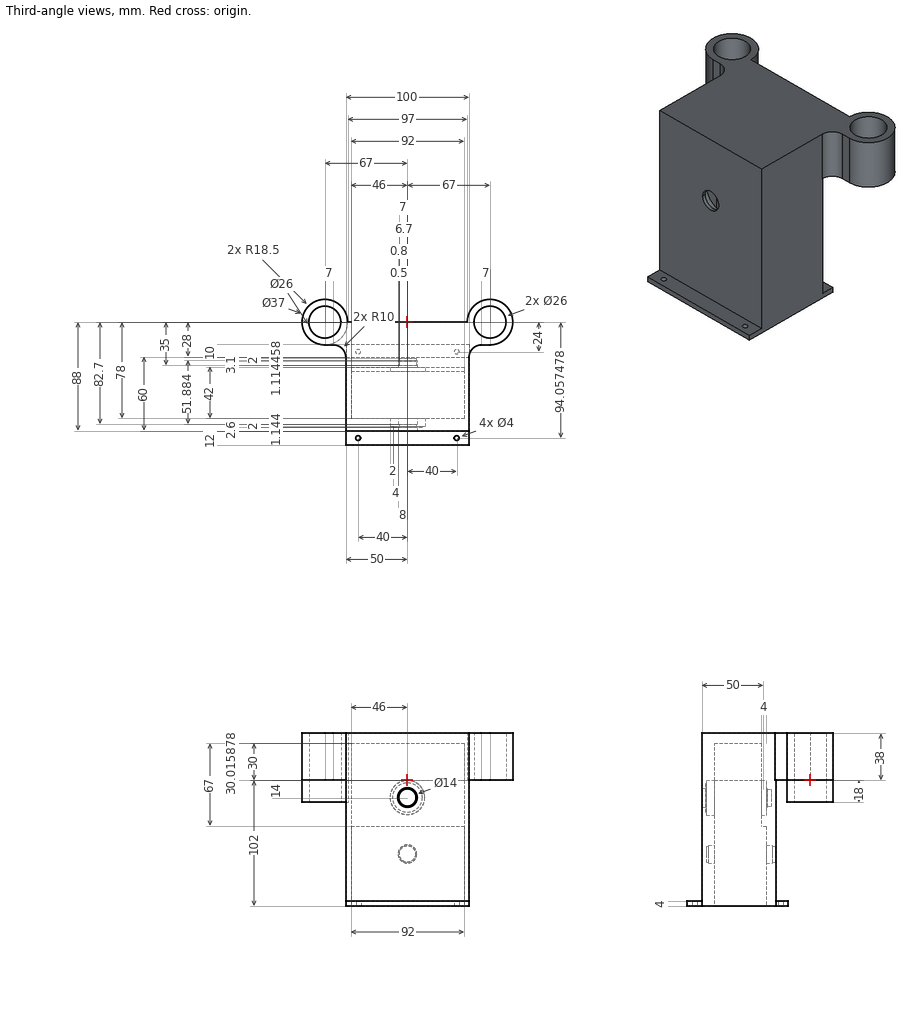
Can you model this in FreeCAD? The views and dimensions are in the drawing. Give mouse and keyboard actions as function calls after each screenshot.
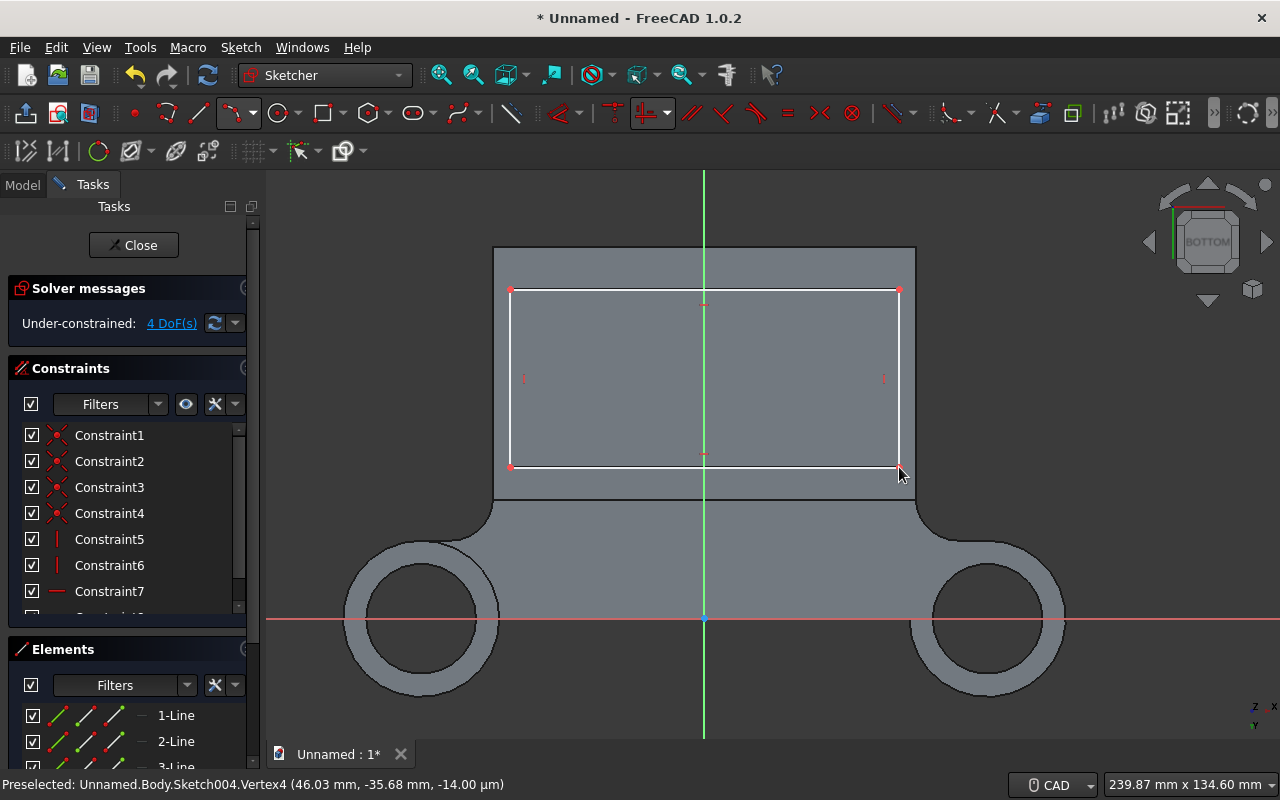
key(d)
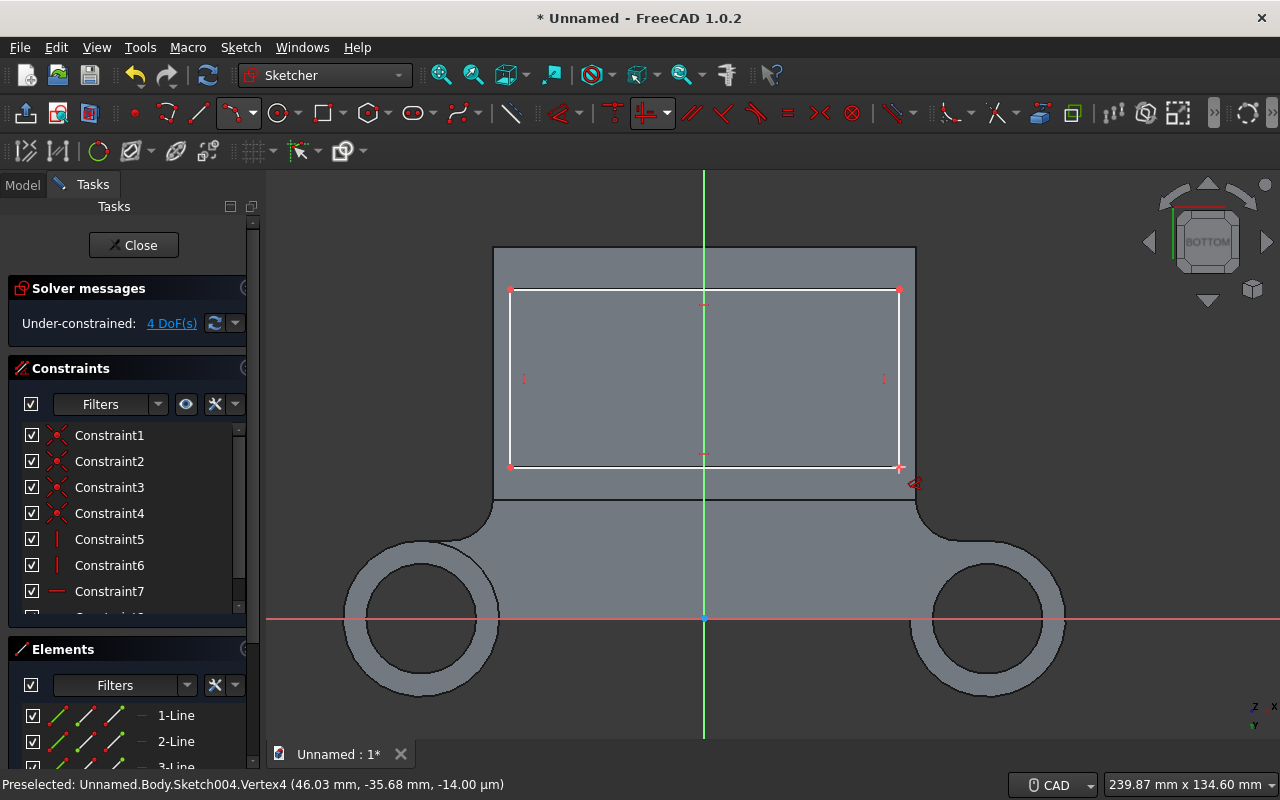
click(510, 343)
click(476, 379)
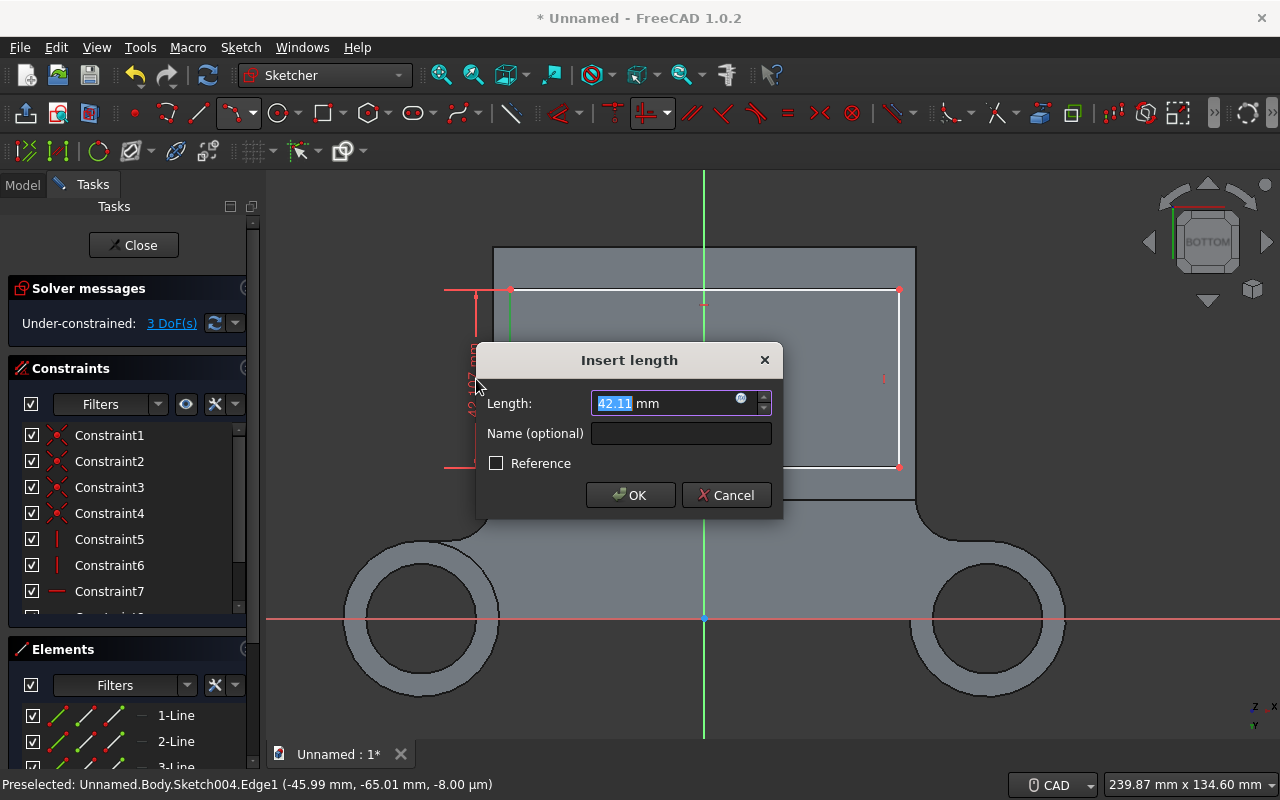
text(42)
key(Return)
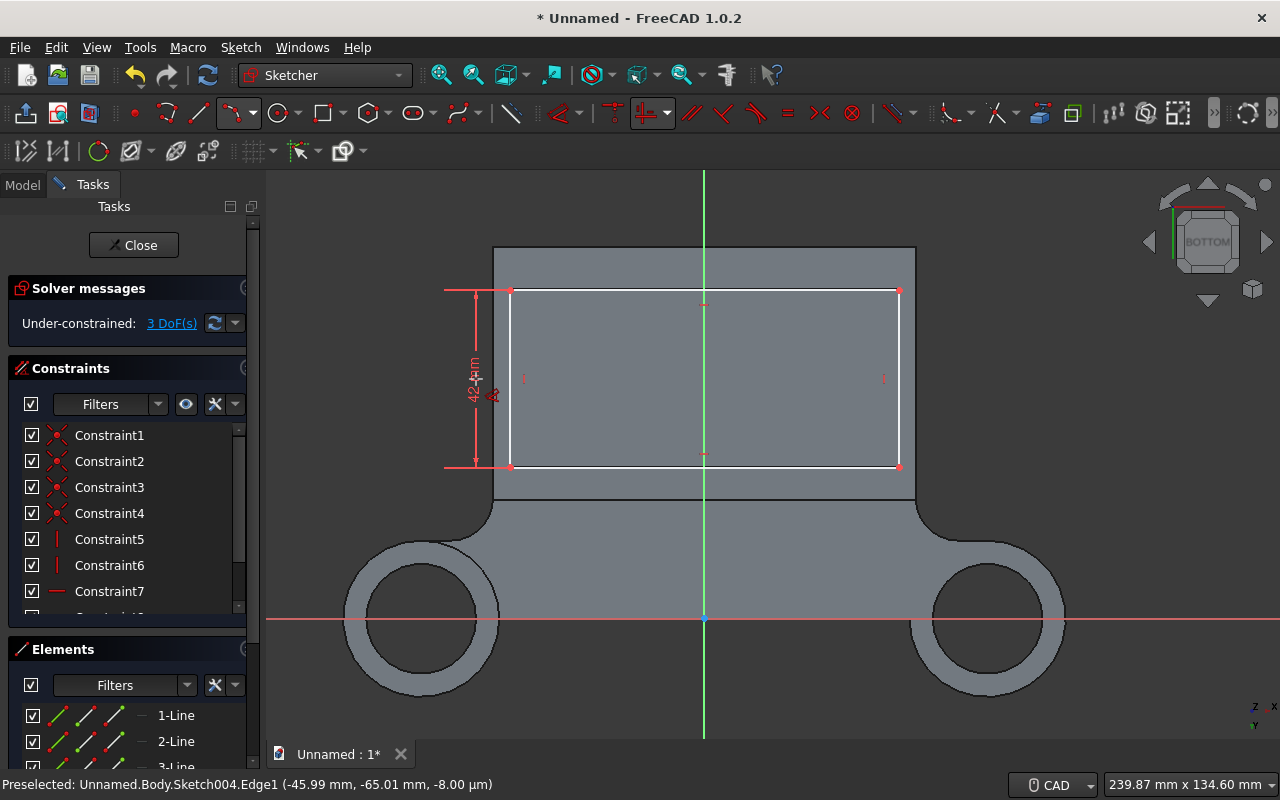
click(627, 468)
click(615, 502)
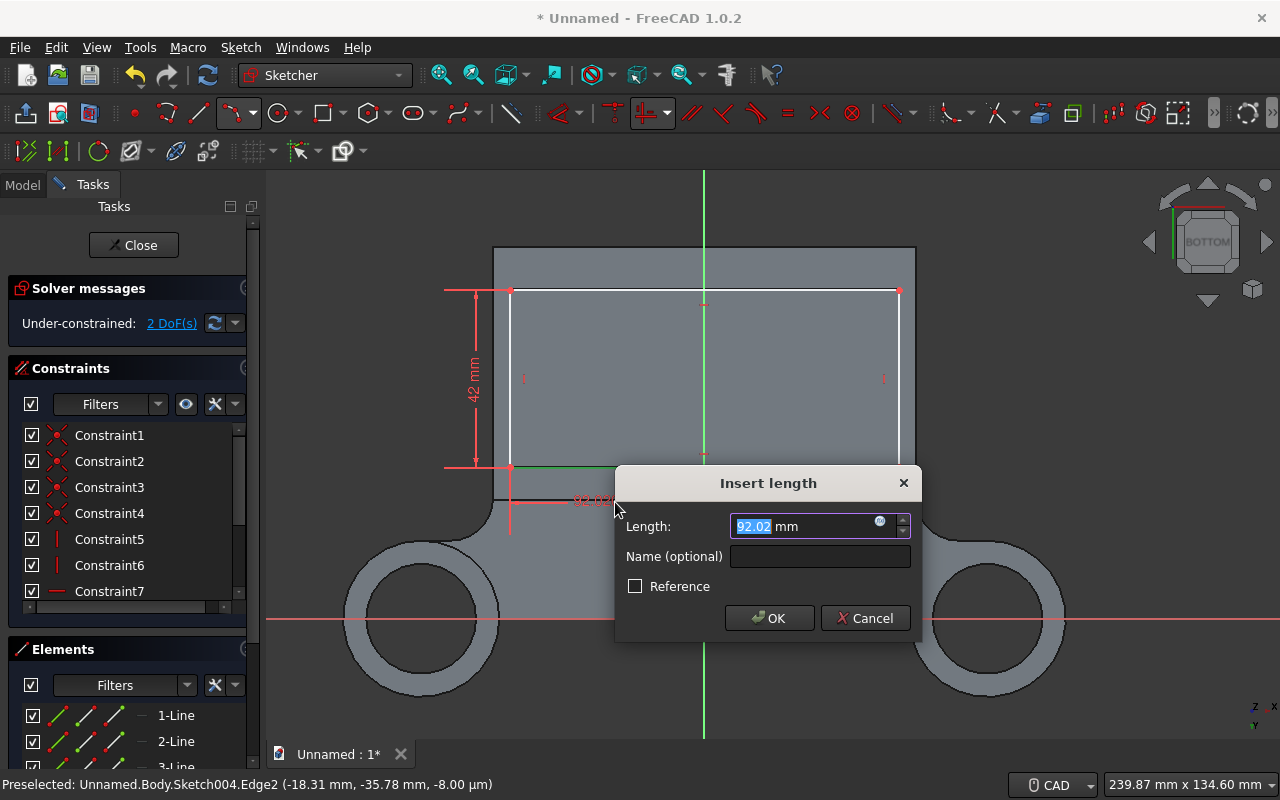
text(92)
key(Return)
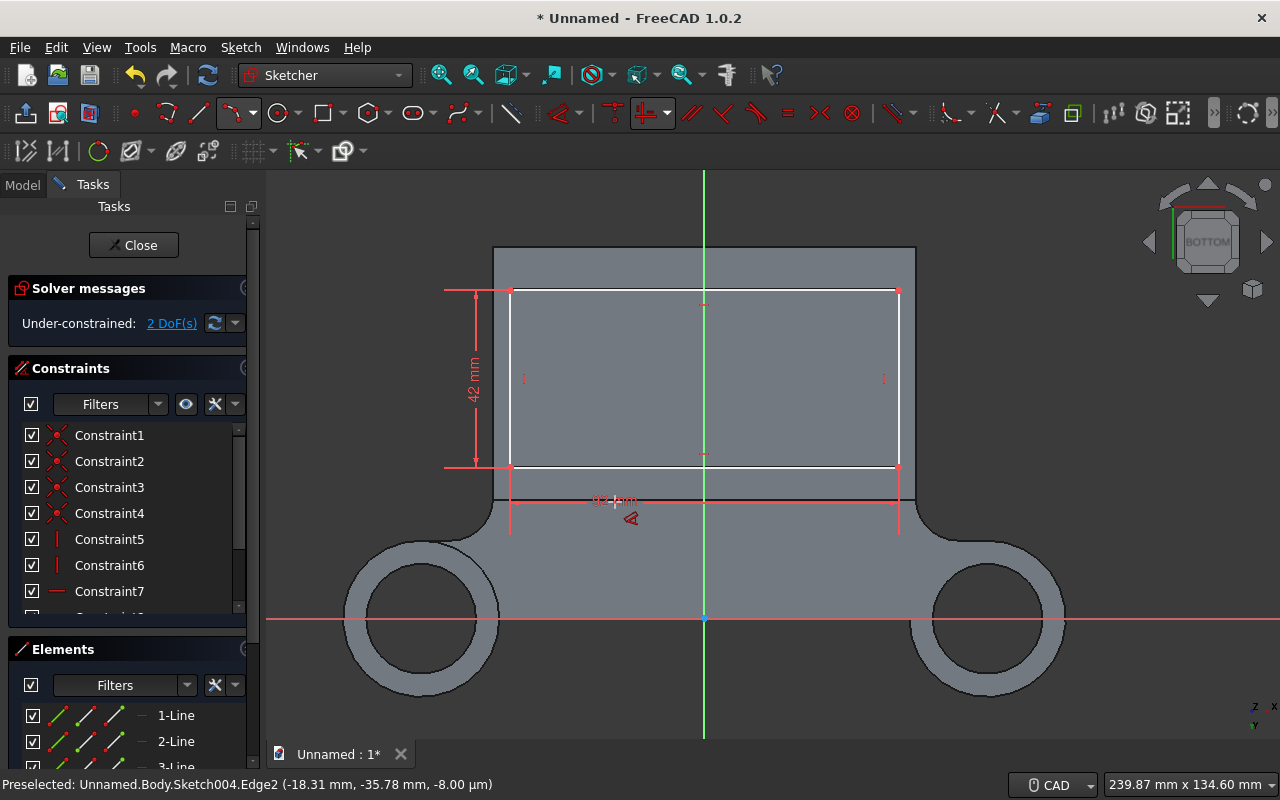
click(510, 290)
click(607, 653)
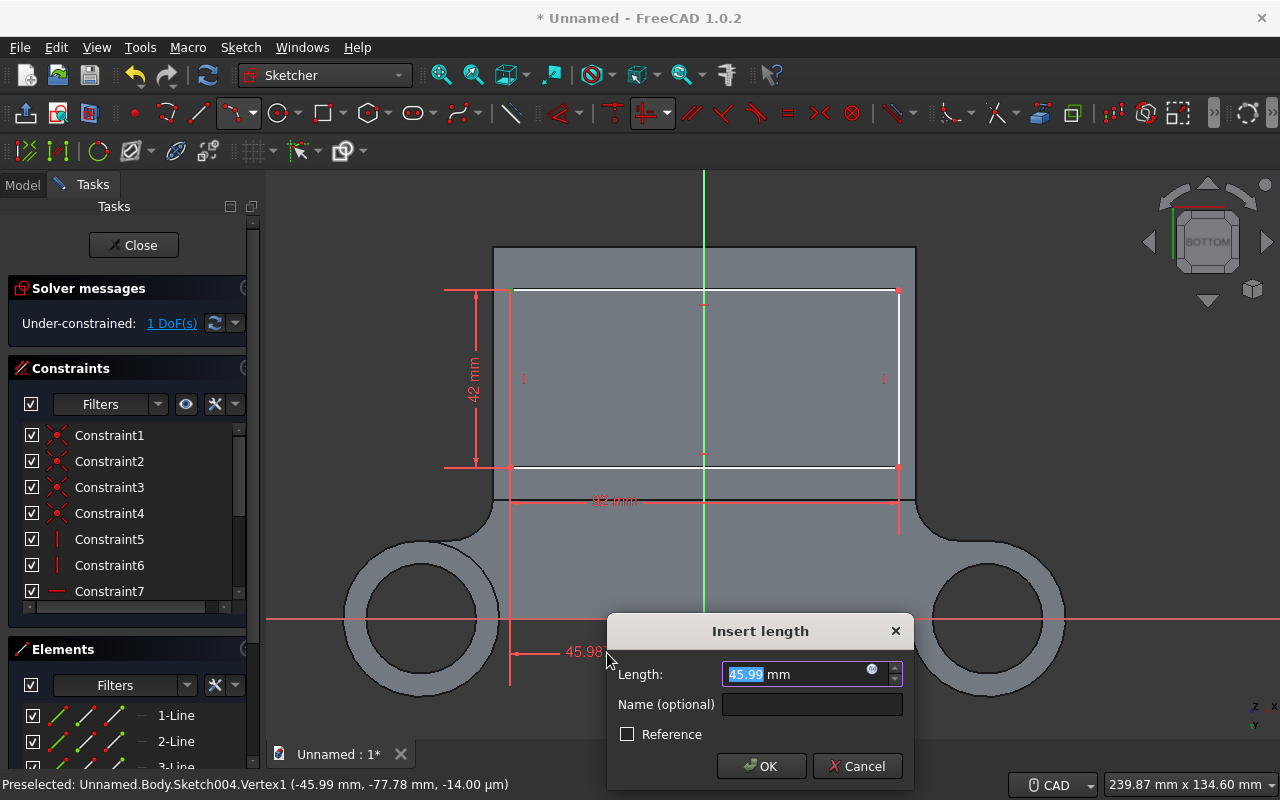
text(46)
key(Return)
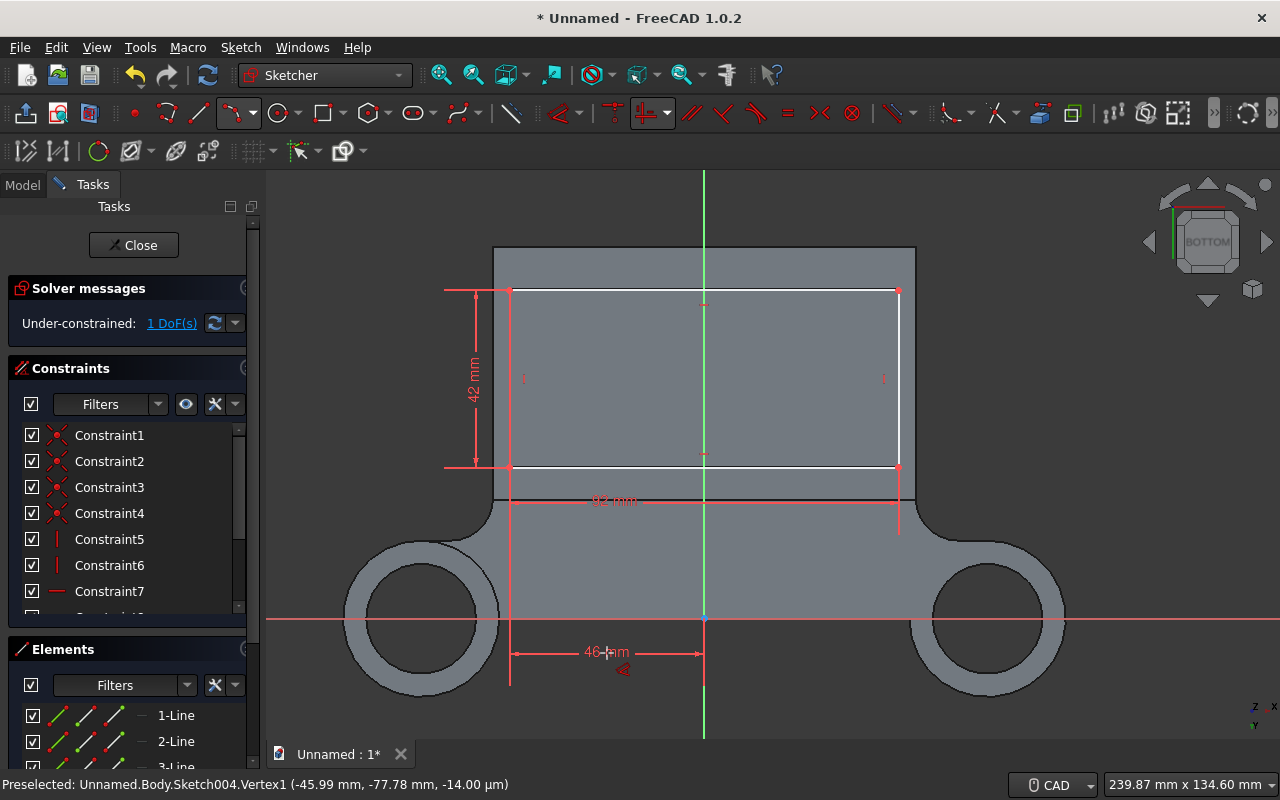
click(510, 290)
click(476, 454)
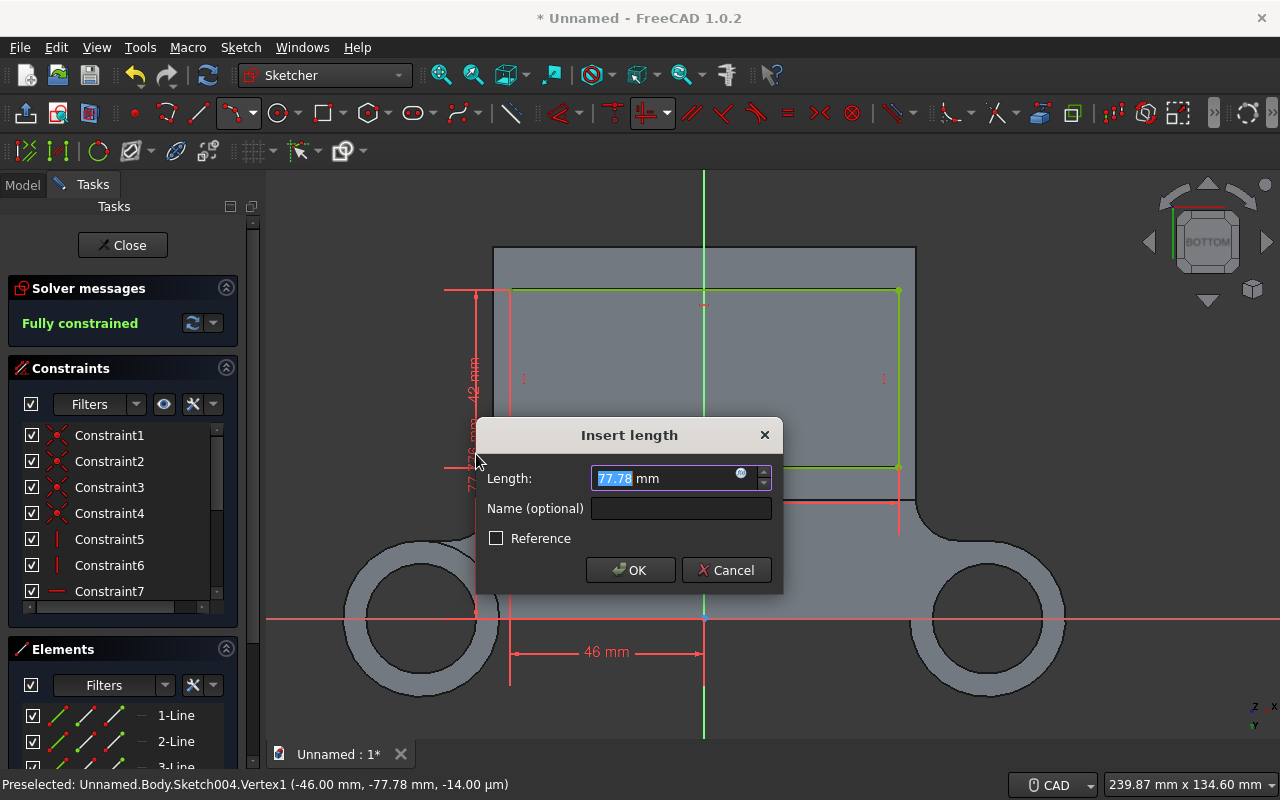
text(78)
key(Return)
key(Escape)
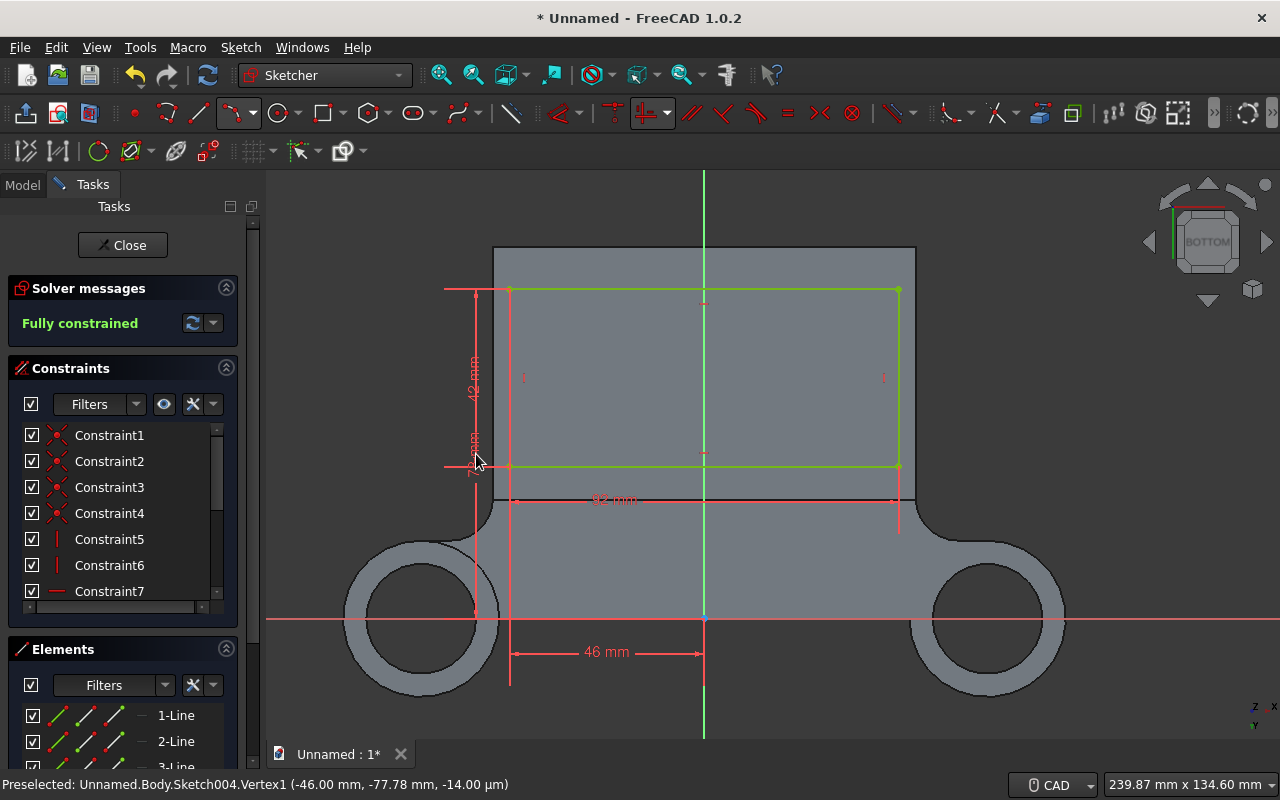
click(123, 245)